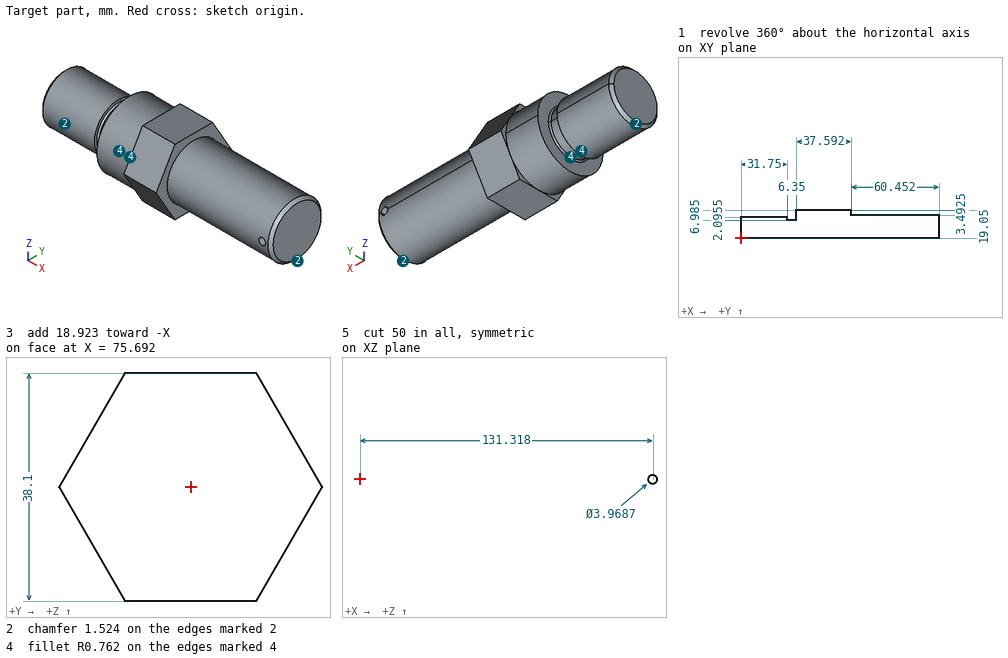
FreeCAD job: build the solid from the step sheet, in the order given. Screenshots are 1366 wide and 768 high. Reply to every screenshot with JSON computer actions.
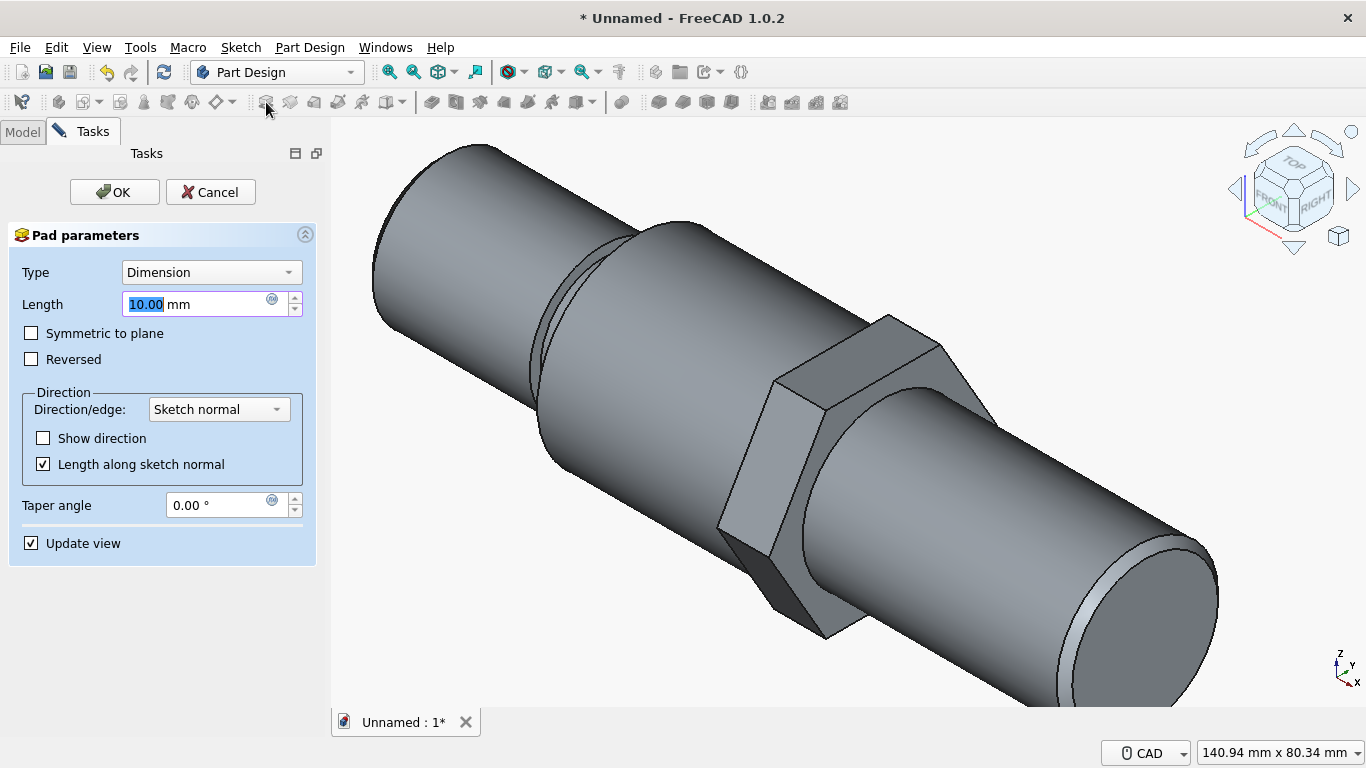
{"action": "type", "text": "18.923"}
{"action": "key", "text": "Tab"}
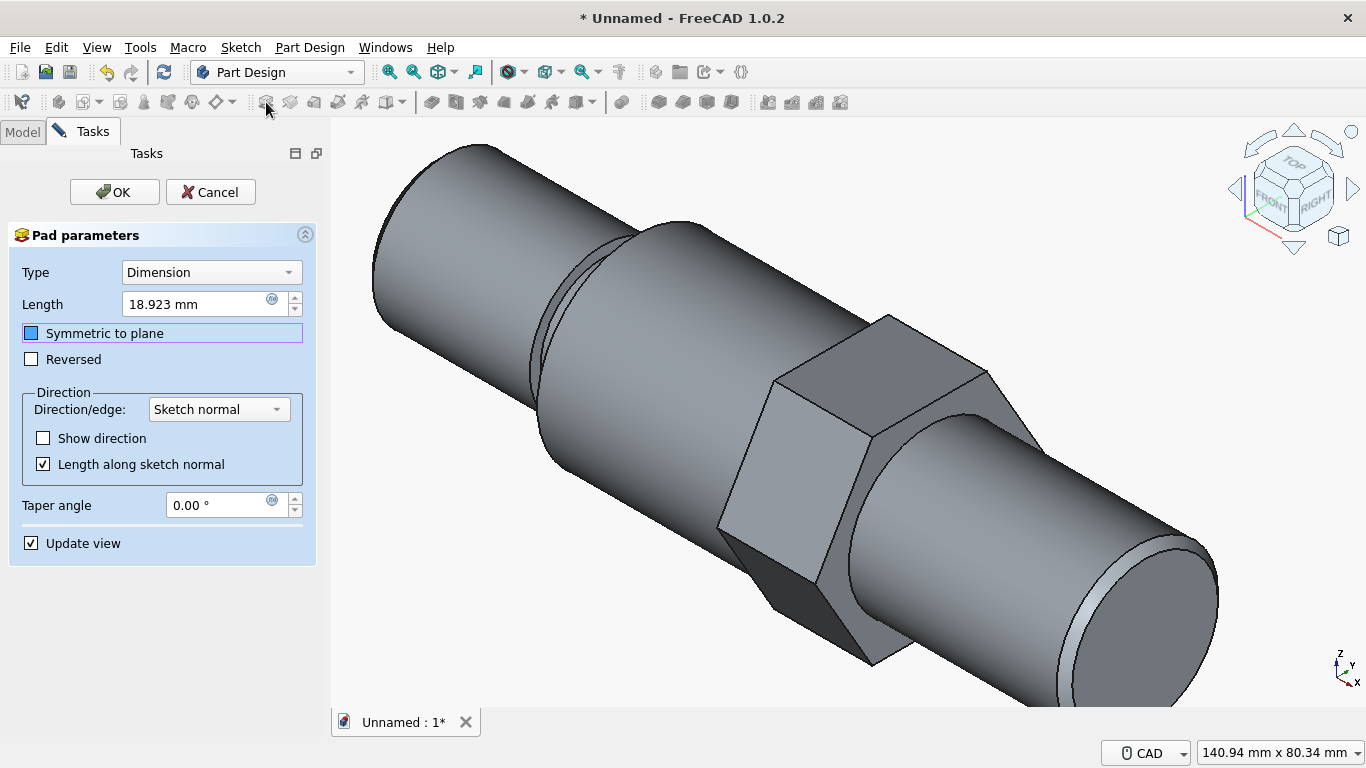
{"action": "left_click", "coordinate": [30, 359]}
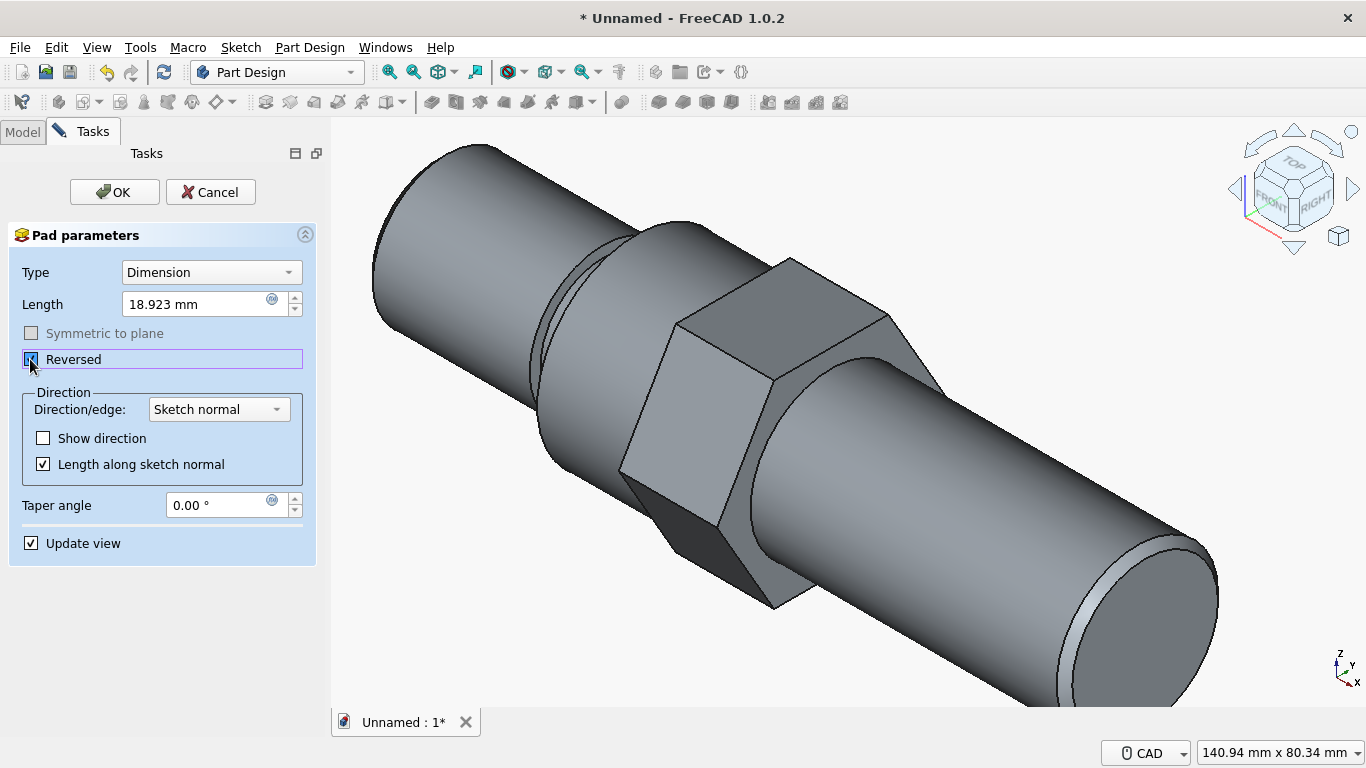
{"action": "left_click", "coordinate": [115, 192]}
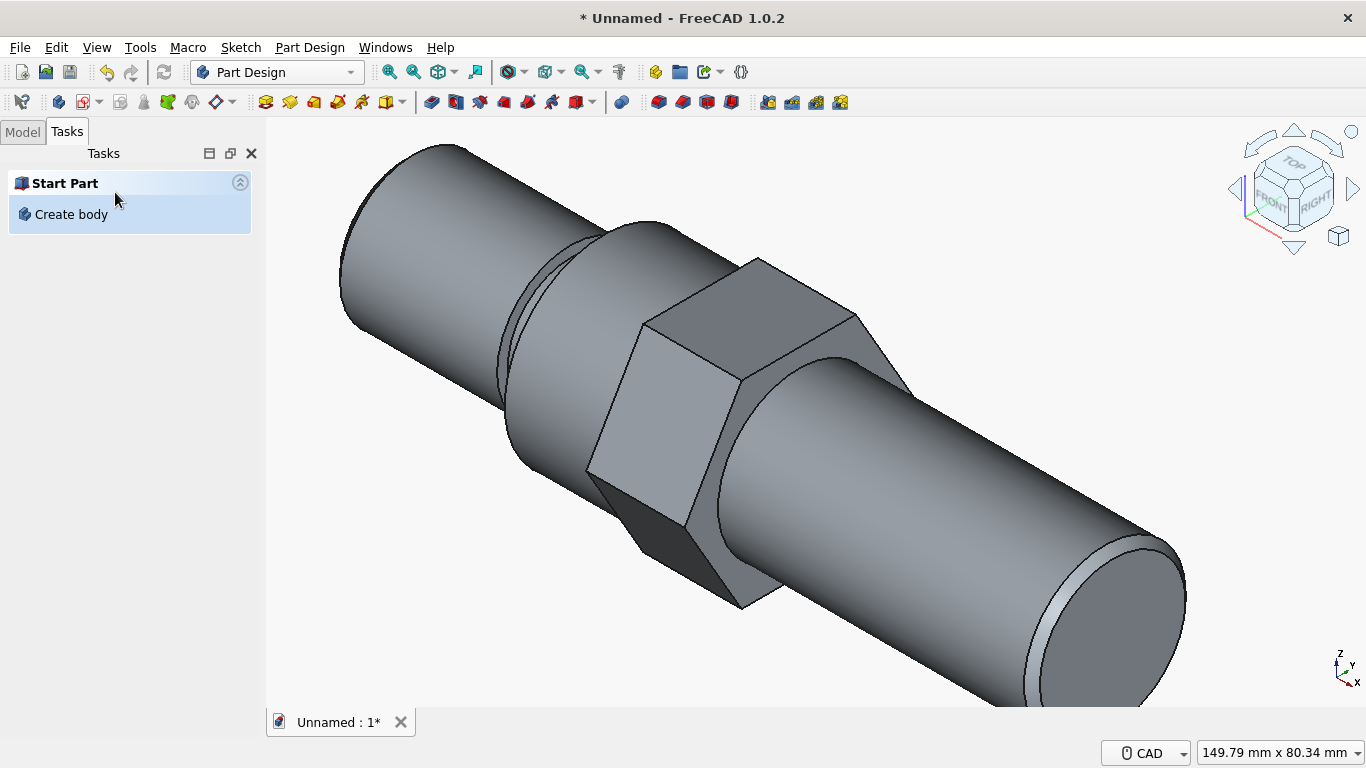
{"action": "key", "text": "v f"}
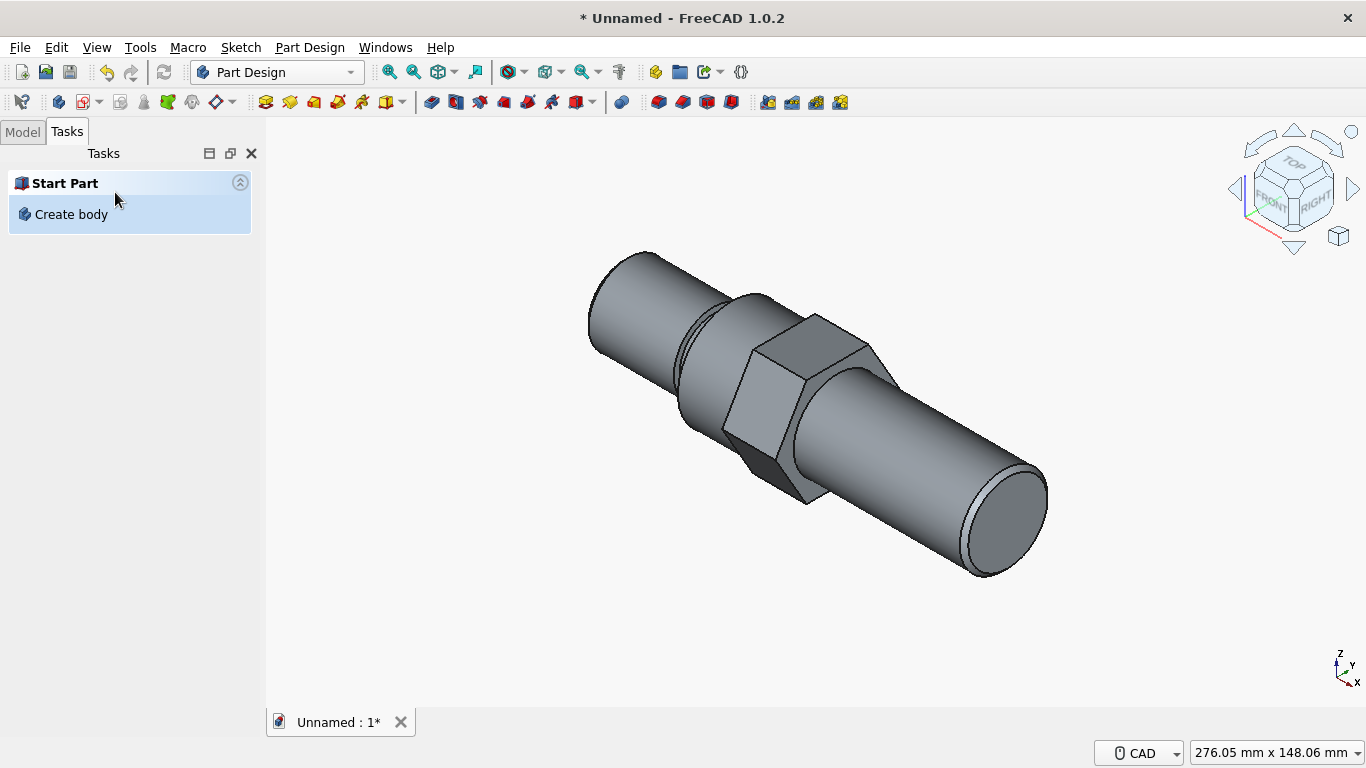
{"action": "key", "text": "2"}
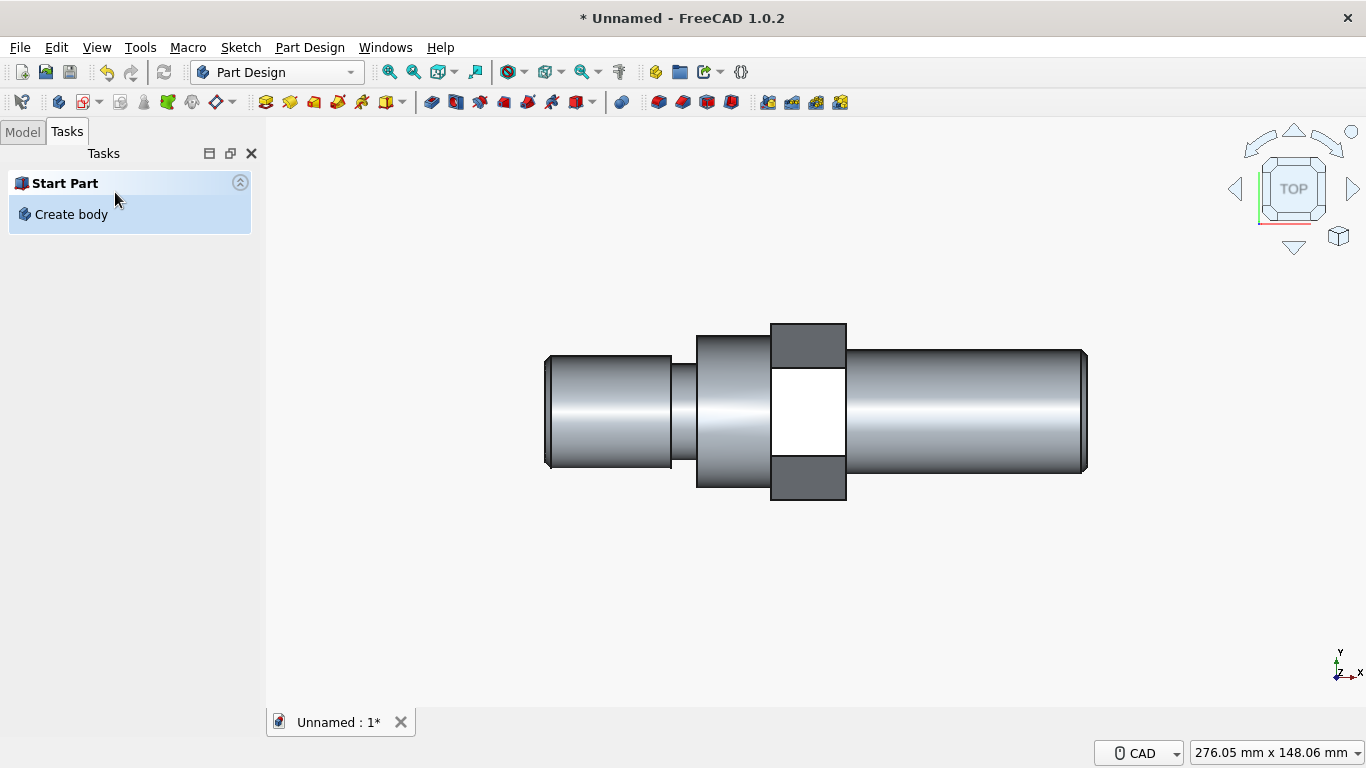
{"action": "key", "text": "0"}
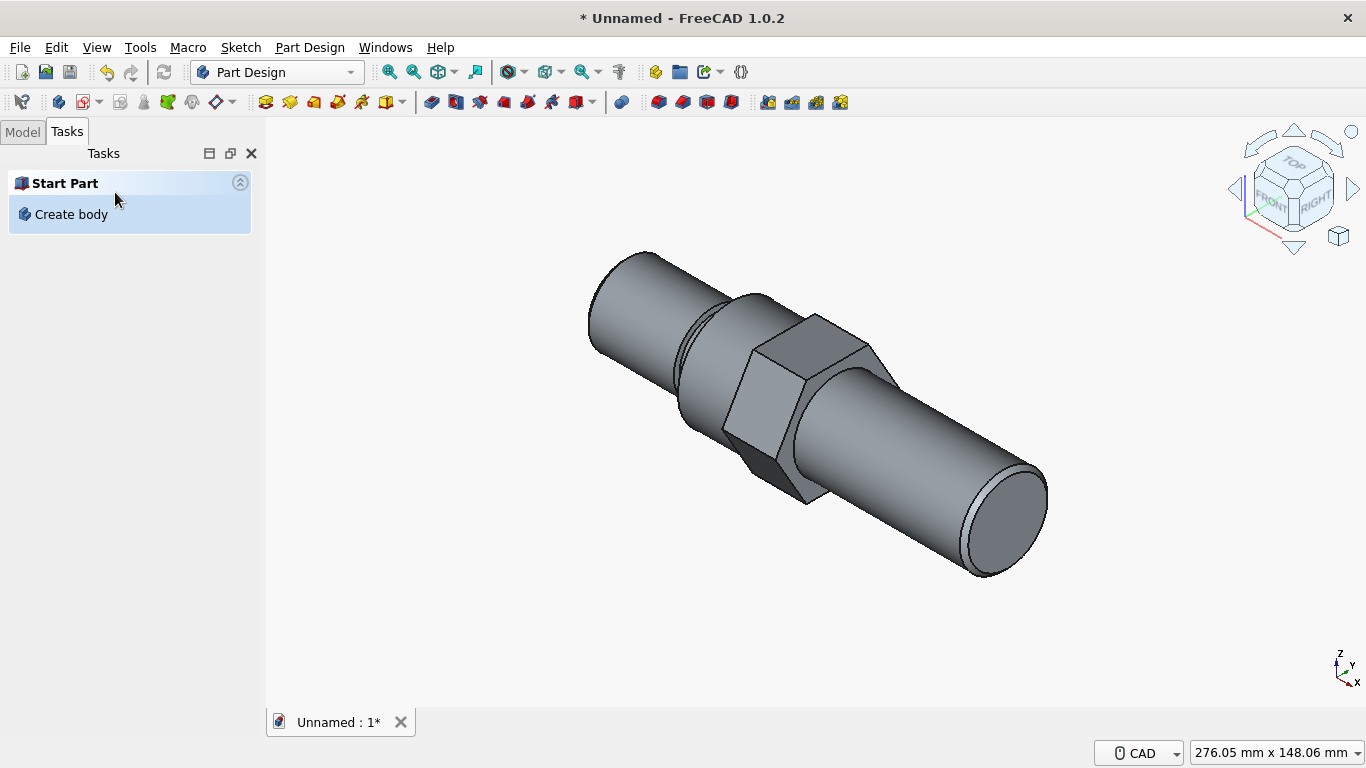
{"action": "key", "text": "1"}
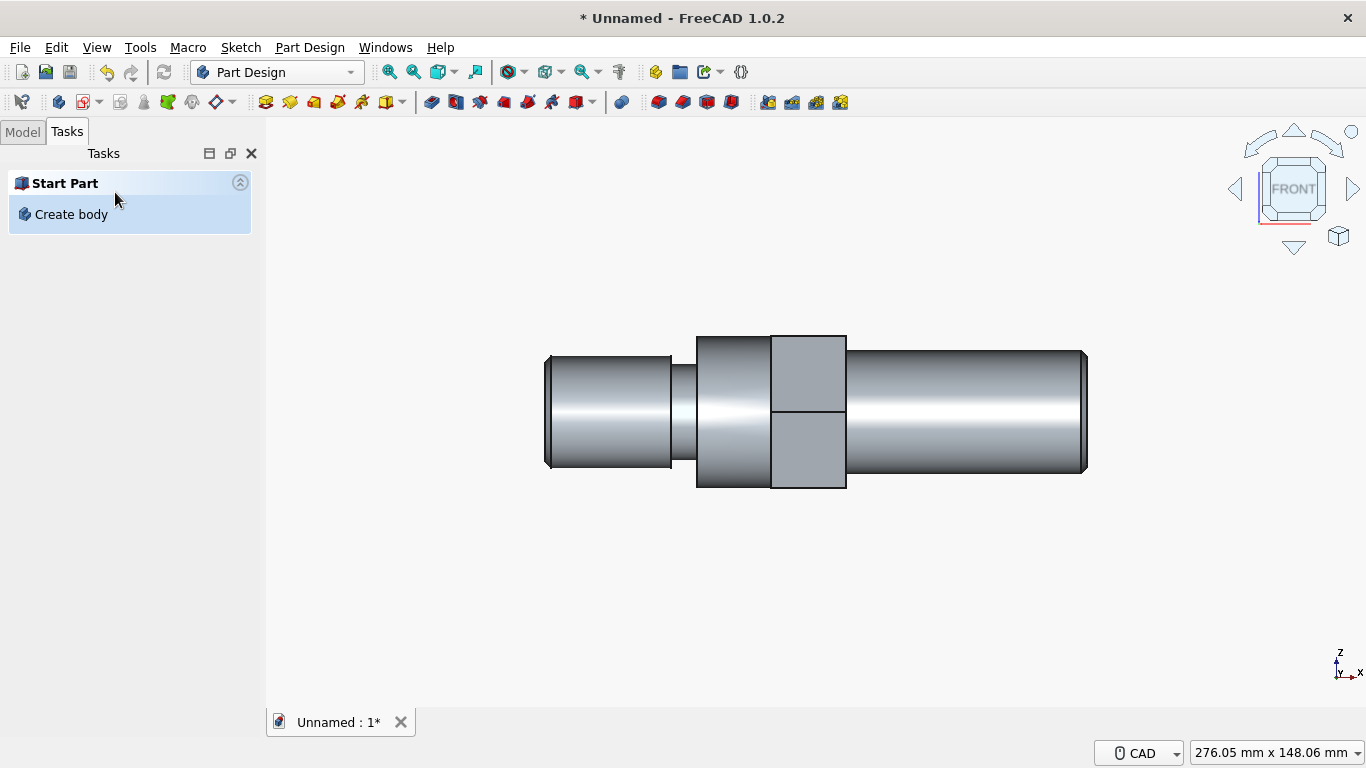
{"action": "key", "text": "3"}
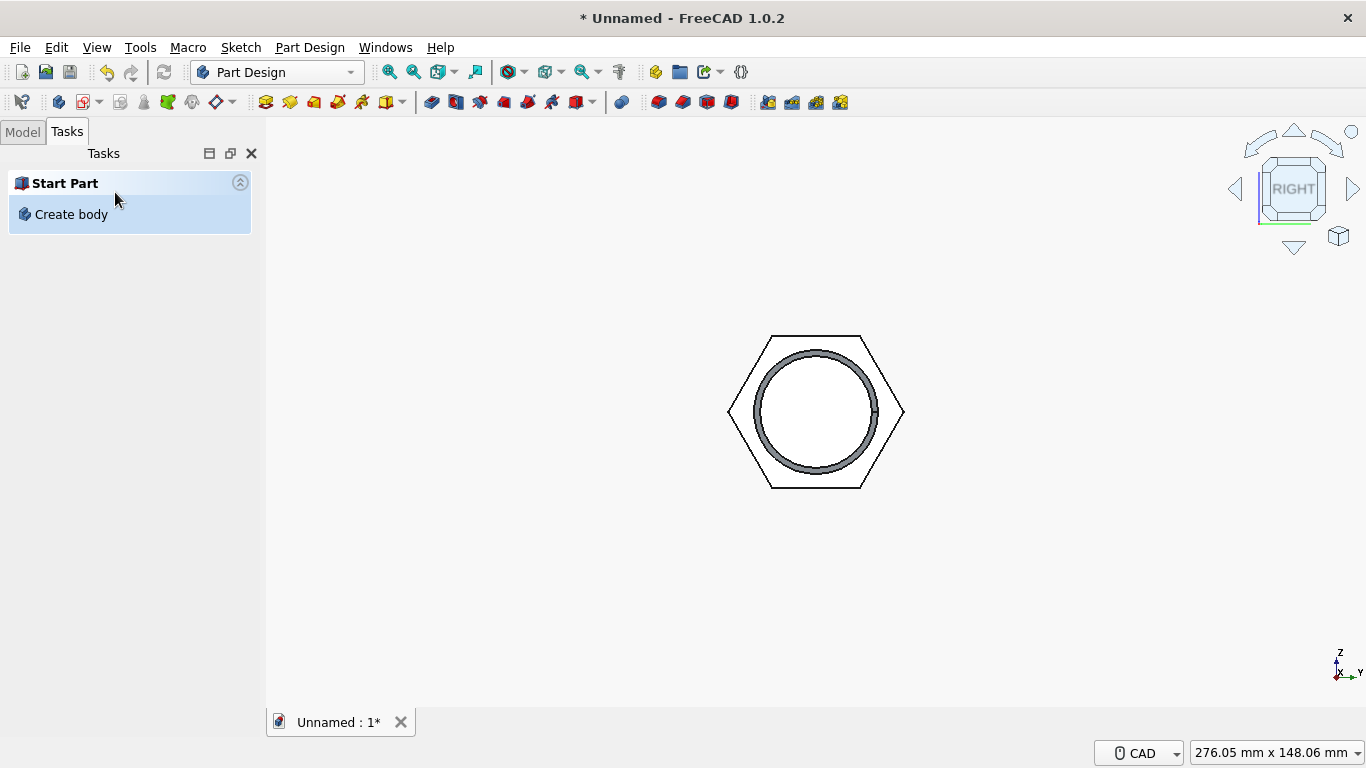
{"action": "key", "text": "v f"}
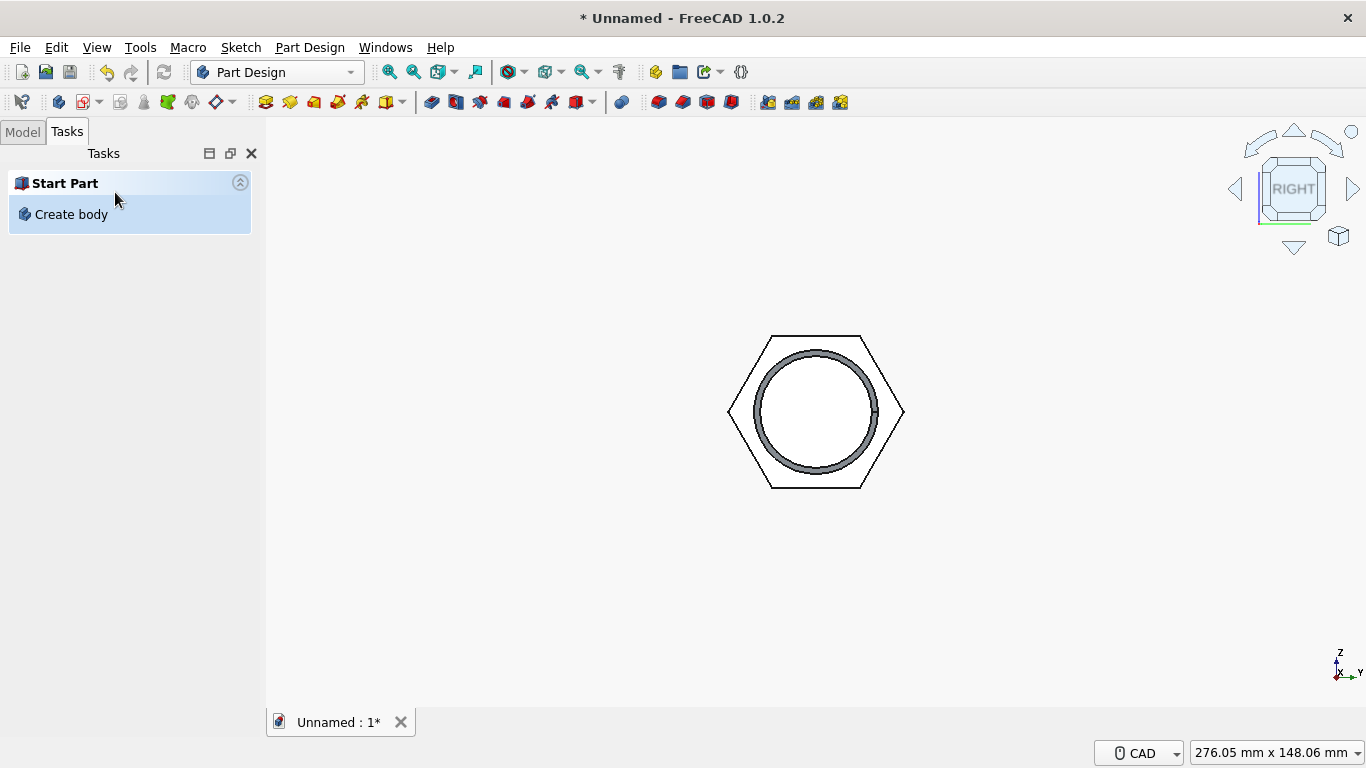
{"action": "key", "text": "5"}